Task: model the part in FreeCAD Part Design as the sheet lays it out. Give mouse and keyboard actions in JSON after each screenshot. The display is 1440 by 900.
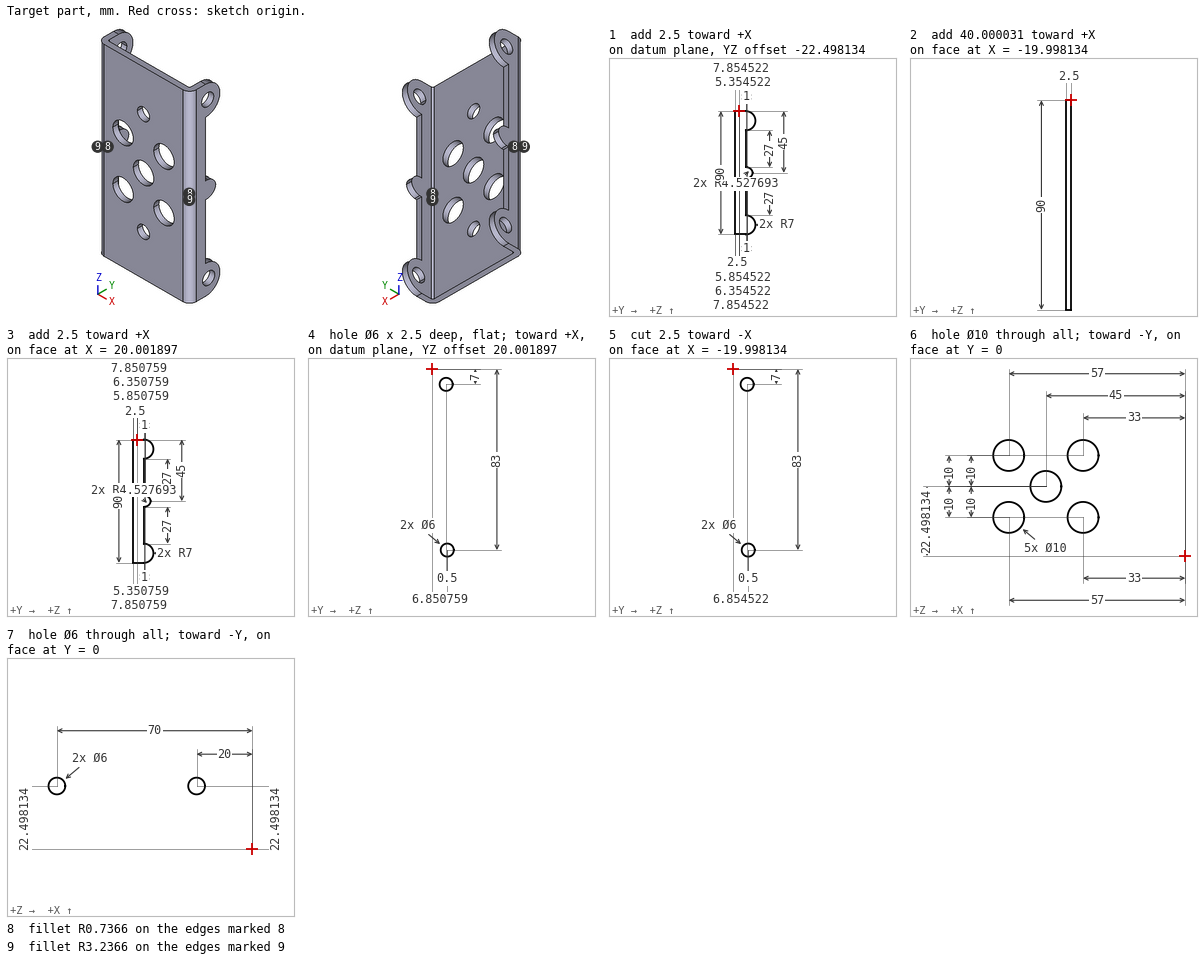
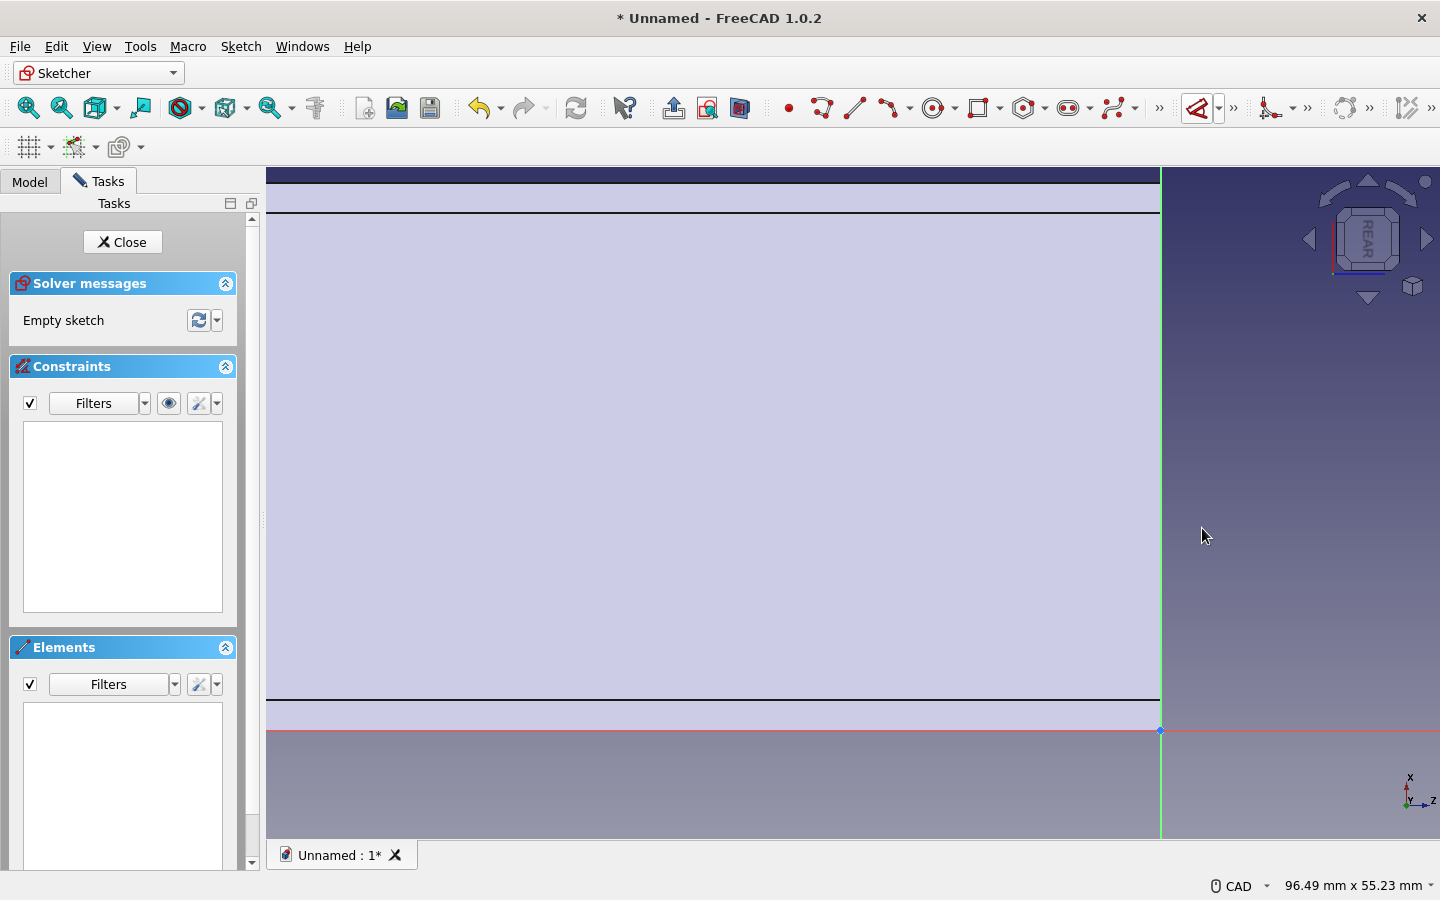
{"action": "key", "text": "g c"}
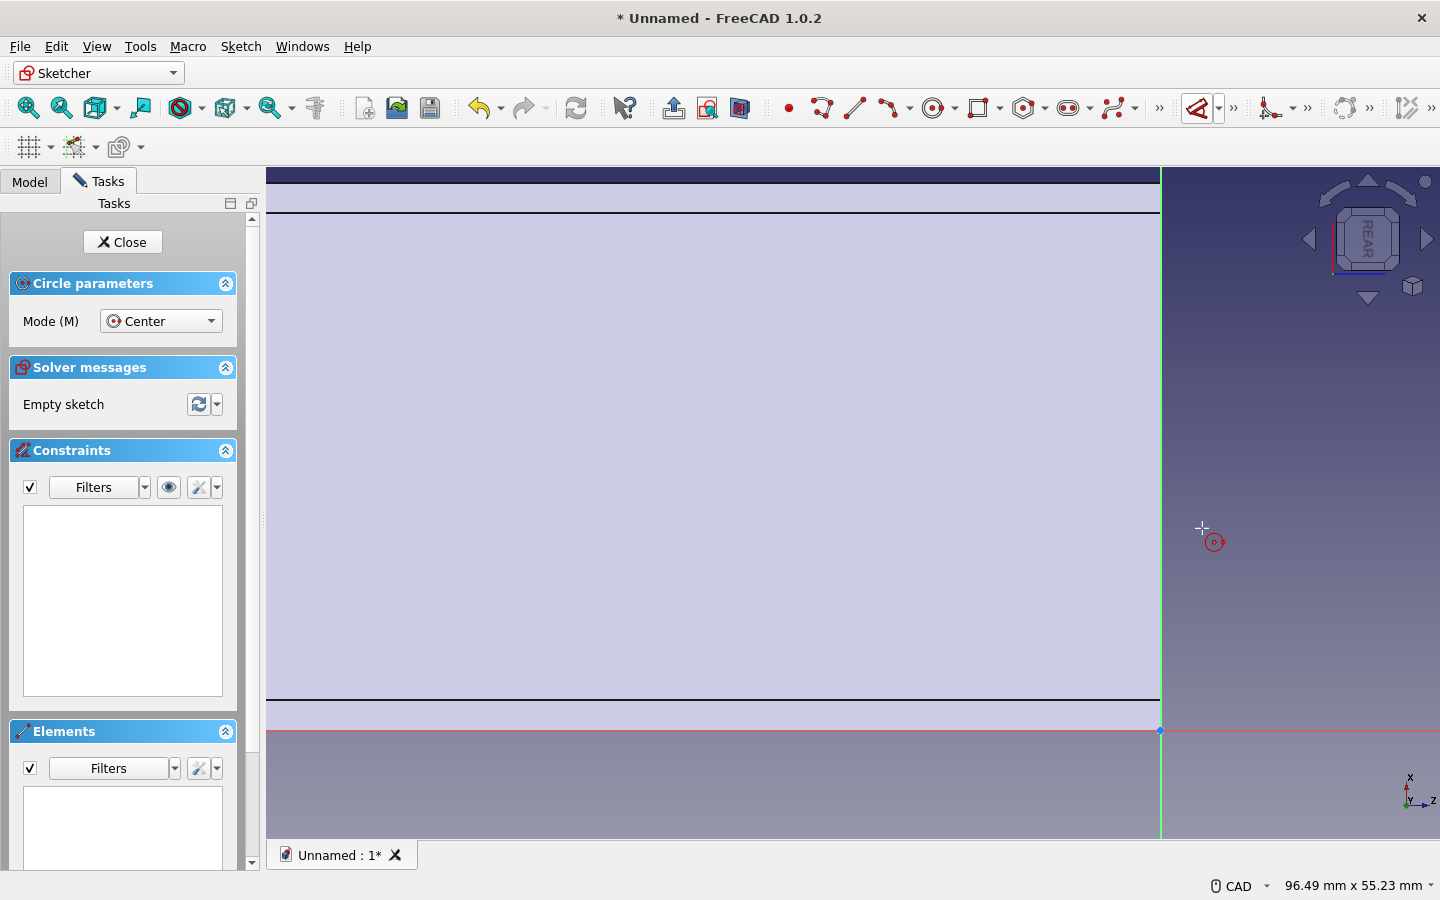
{"action": "left_click", "coordinate": [613, 457]}
{"action": "mouse_move", "coordinate": [656, 414]}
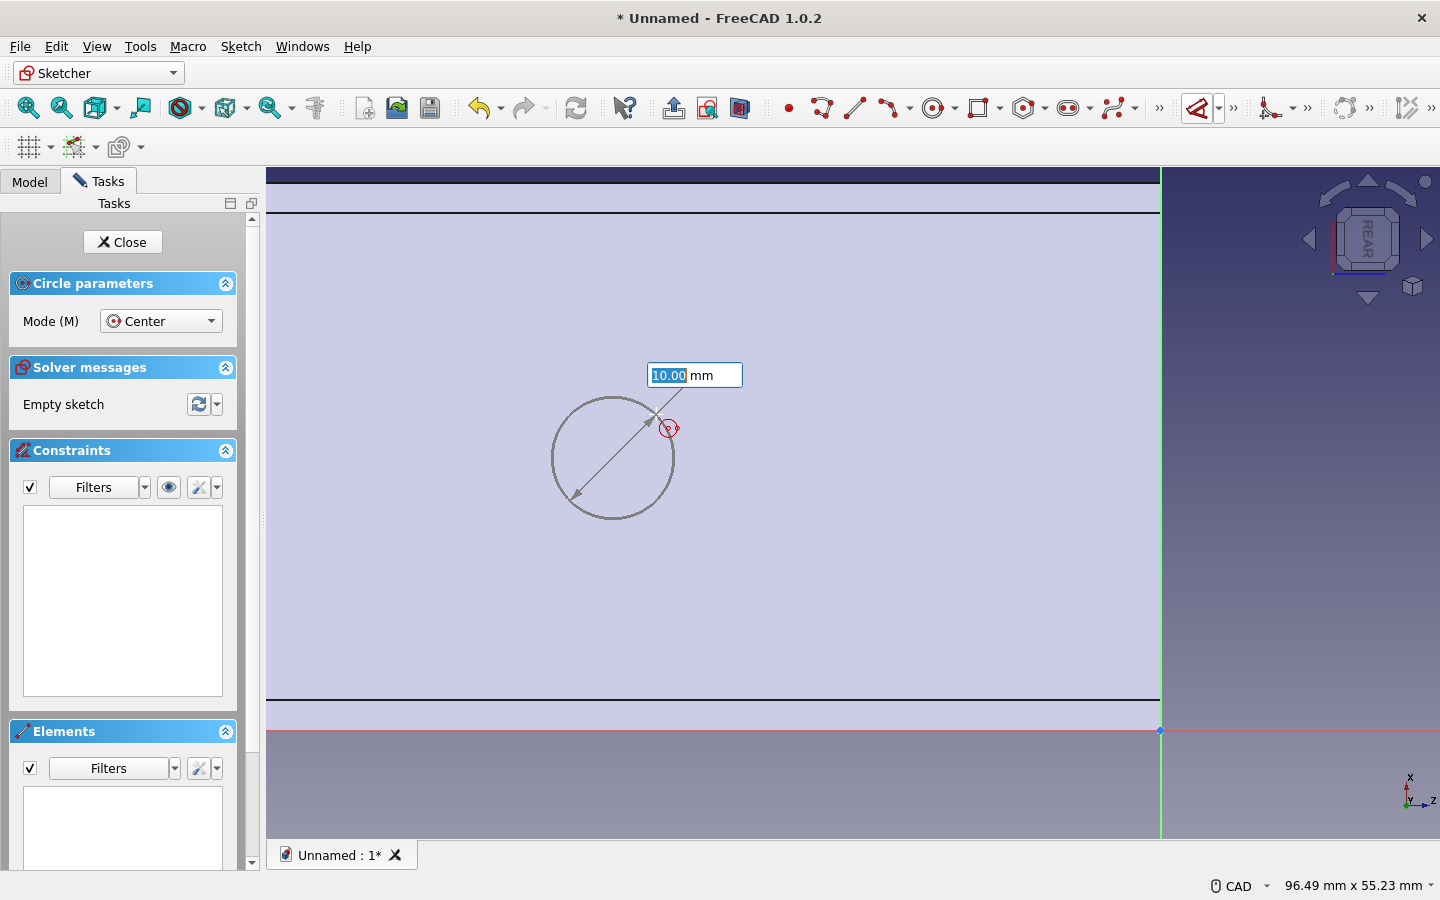
{"action": "type", "text": "10"}
{"action": "key", "text": "Return"}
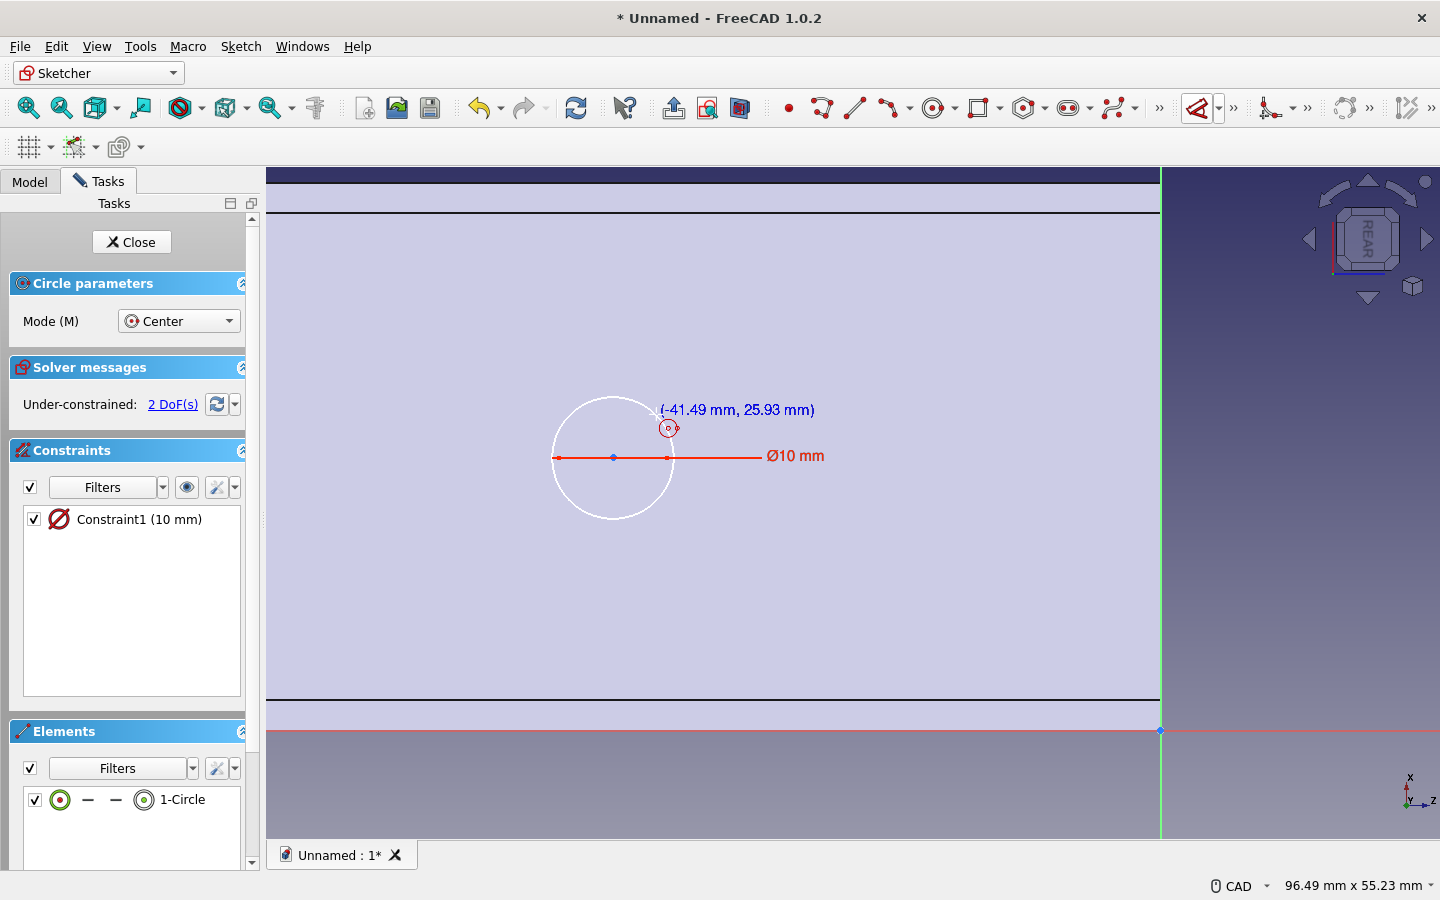
{"action": "left_click", "coordinate": [467, 578]}
{"action": "mouse_move", "coordinate": [510, 535]}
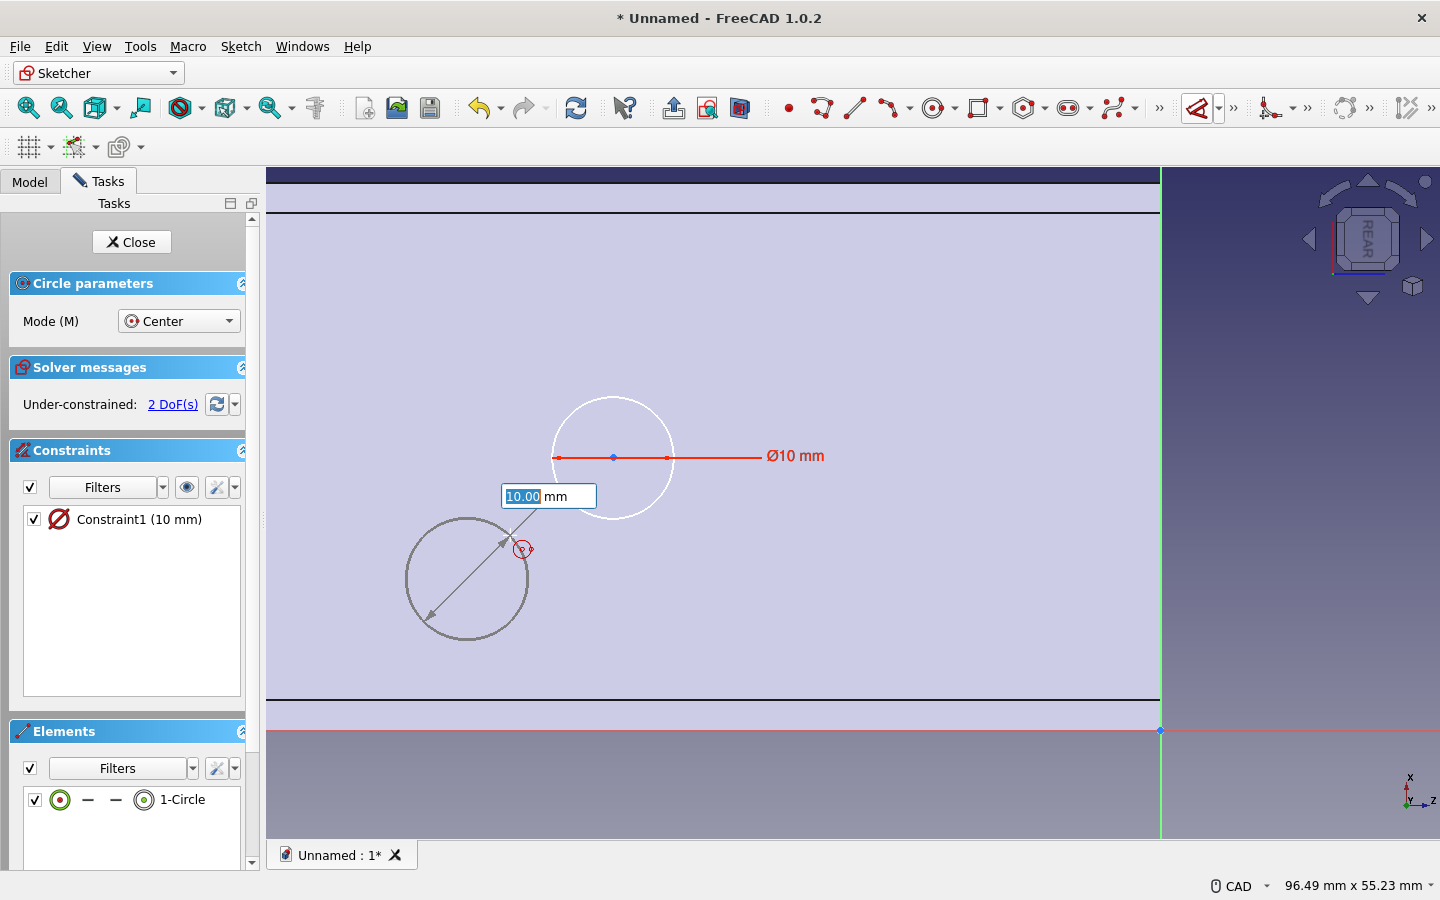
{"action": "type", "text": "10"}
{"action": "key", "text": "Return"}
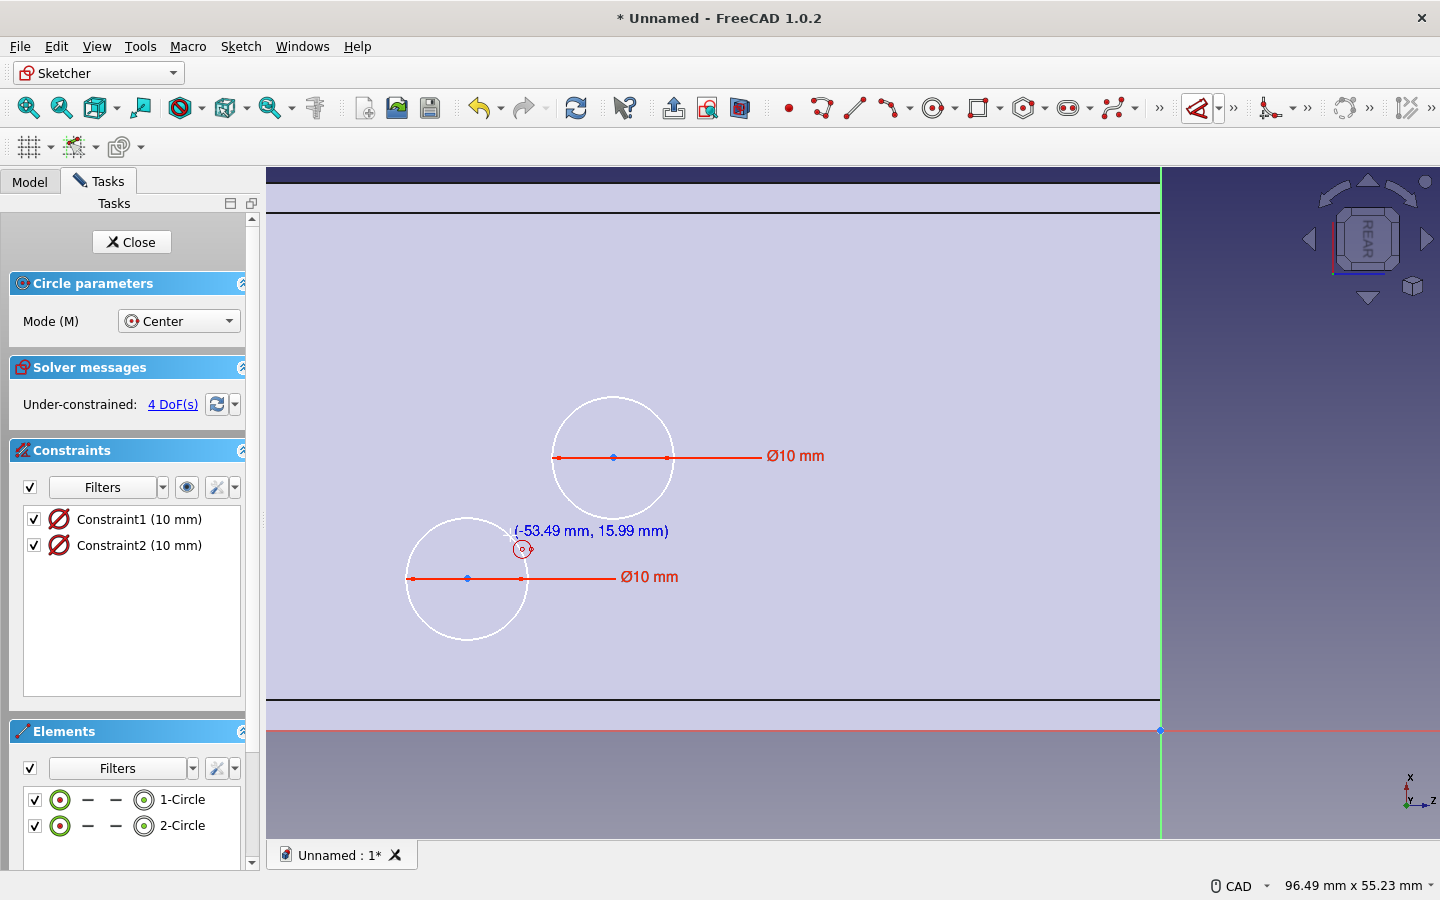
{"action": "left_click", "coordinate": [759, 578]}
{"action": "mouse_move", "coordinate": [802, 535]}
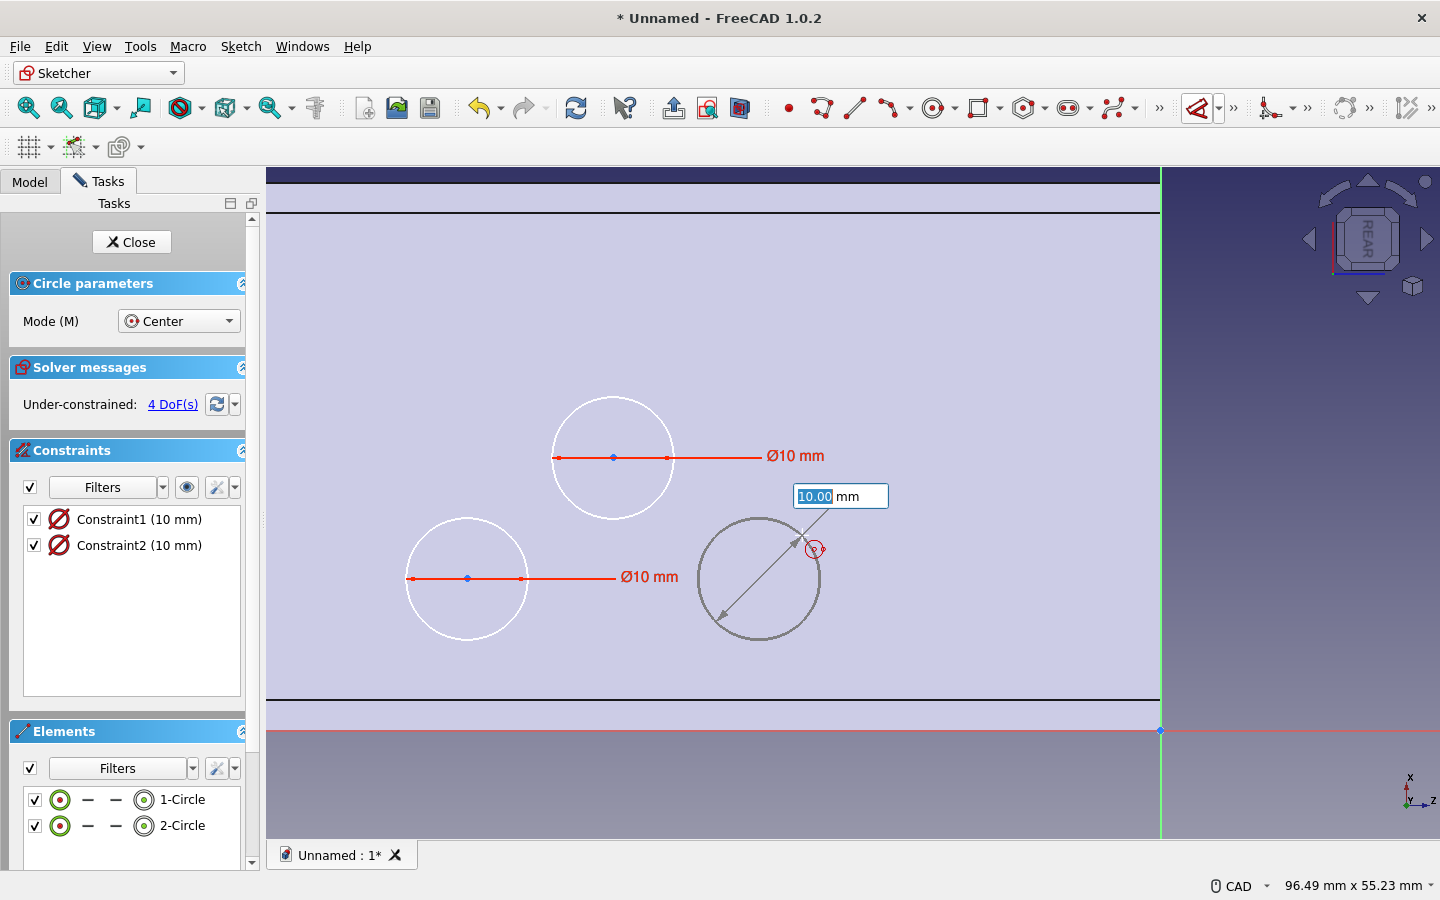
{"action": "type", "text": "10"}
{"action": "key", "text": "Return"}